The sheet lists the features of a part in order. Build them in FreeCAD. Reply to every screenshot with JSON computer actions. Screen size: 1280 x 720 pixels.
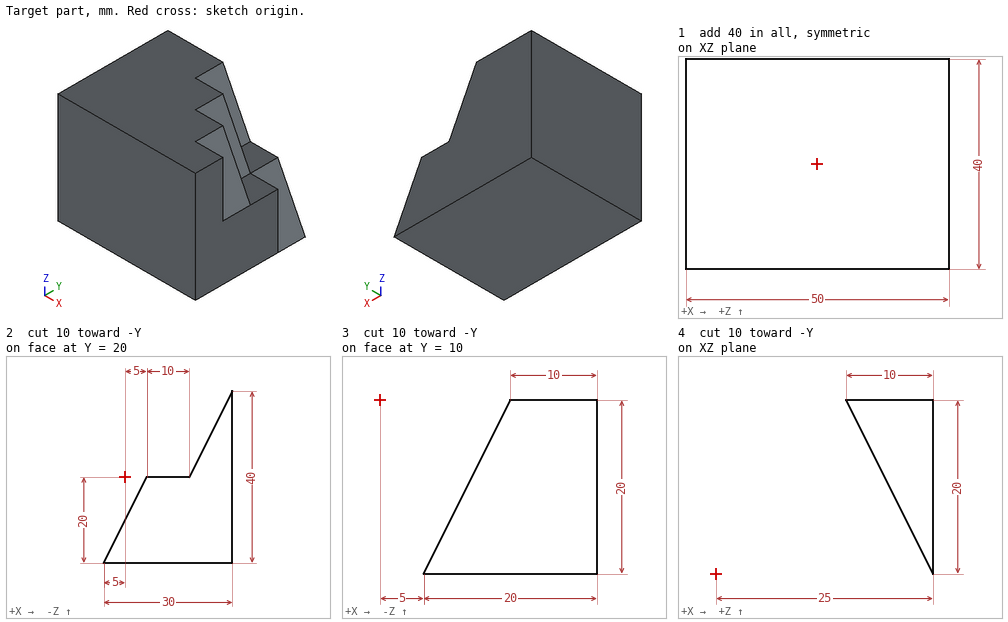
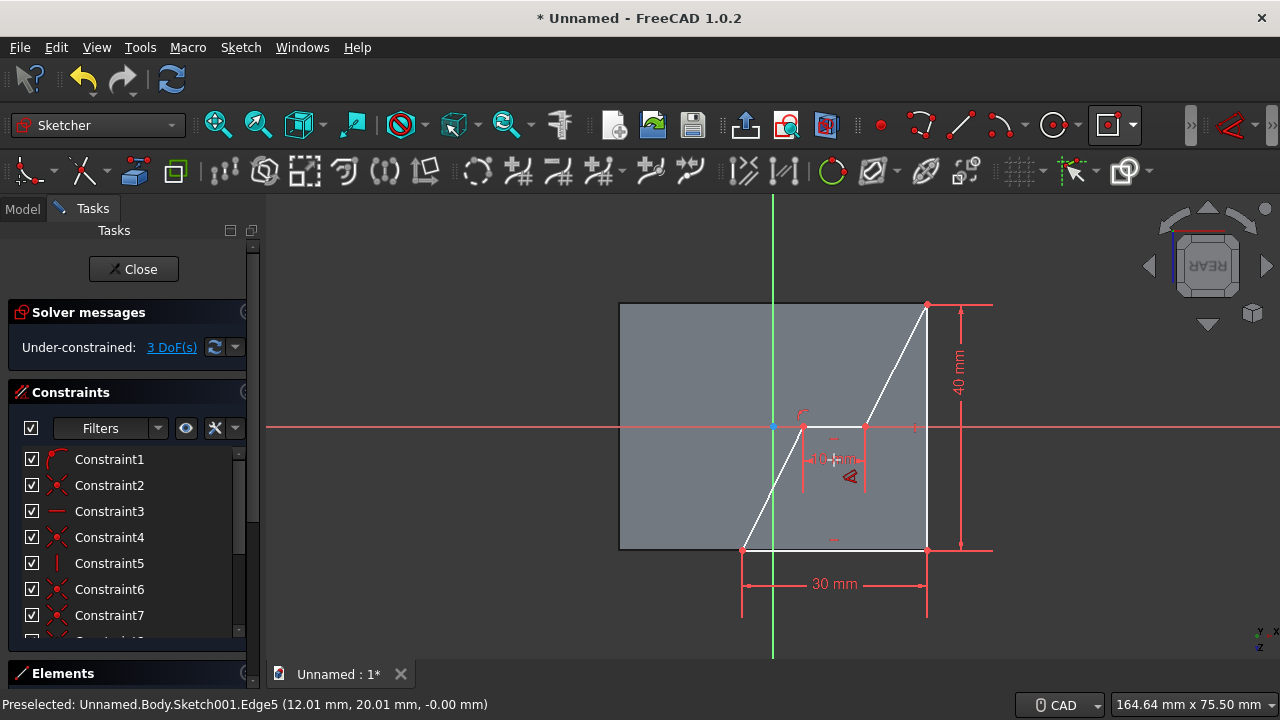
{"action": "scroll", "coordinate": [803, 426], "scroll_direction": "up", "scroll_amount": 2}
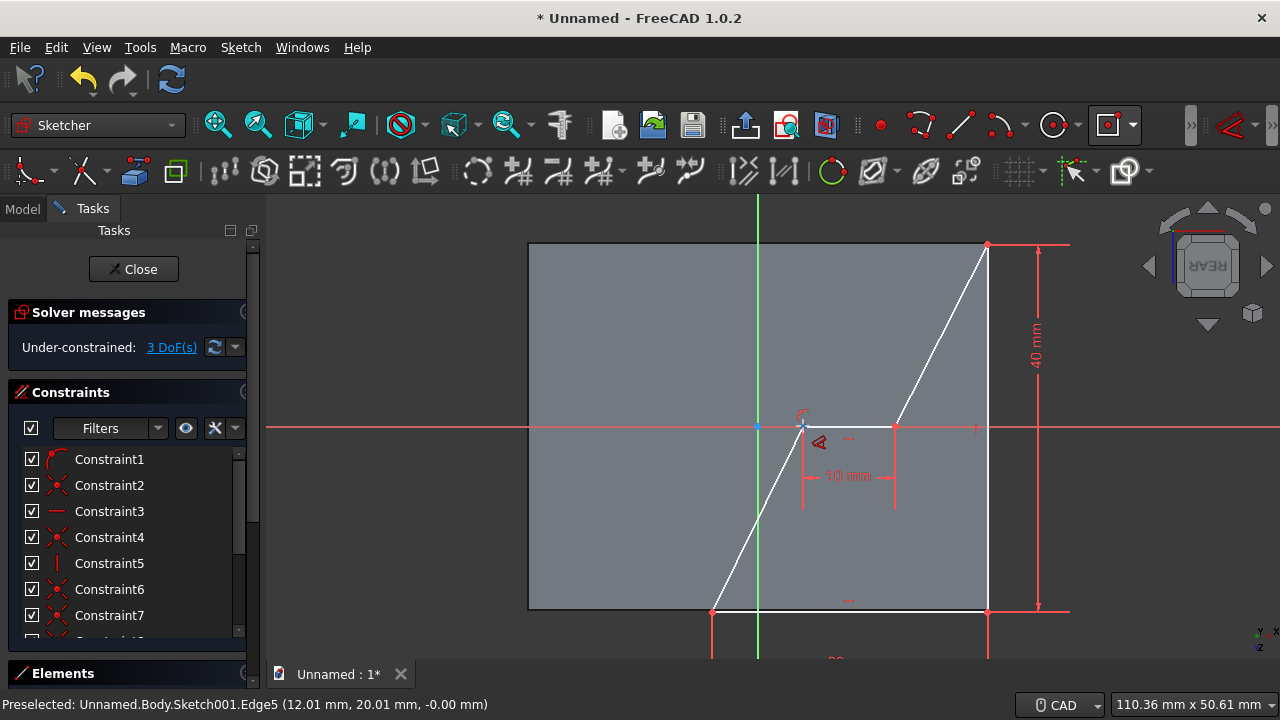
{"action": "left_click", "coordinate": [803, 426]}
{"action": "left_click", "coordinate": [781, 392]}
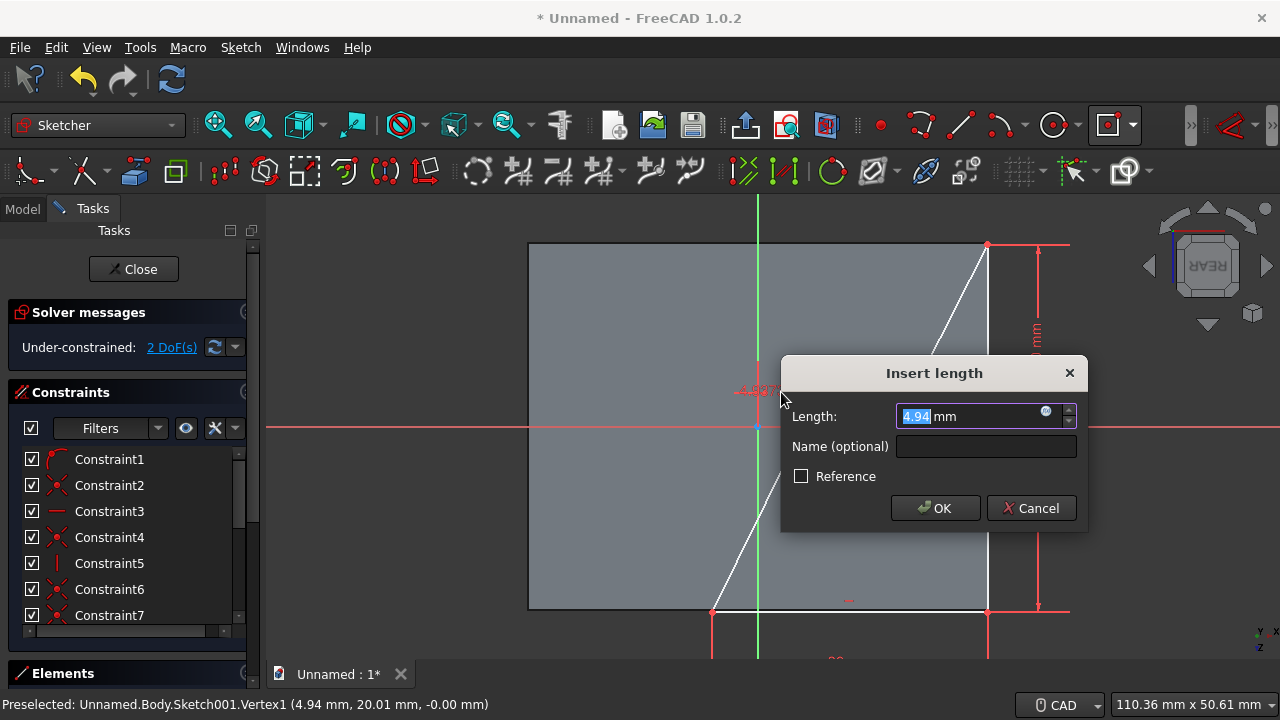
{"action": "type", "text": "5"}
{"action": "key", "text": "Return"}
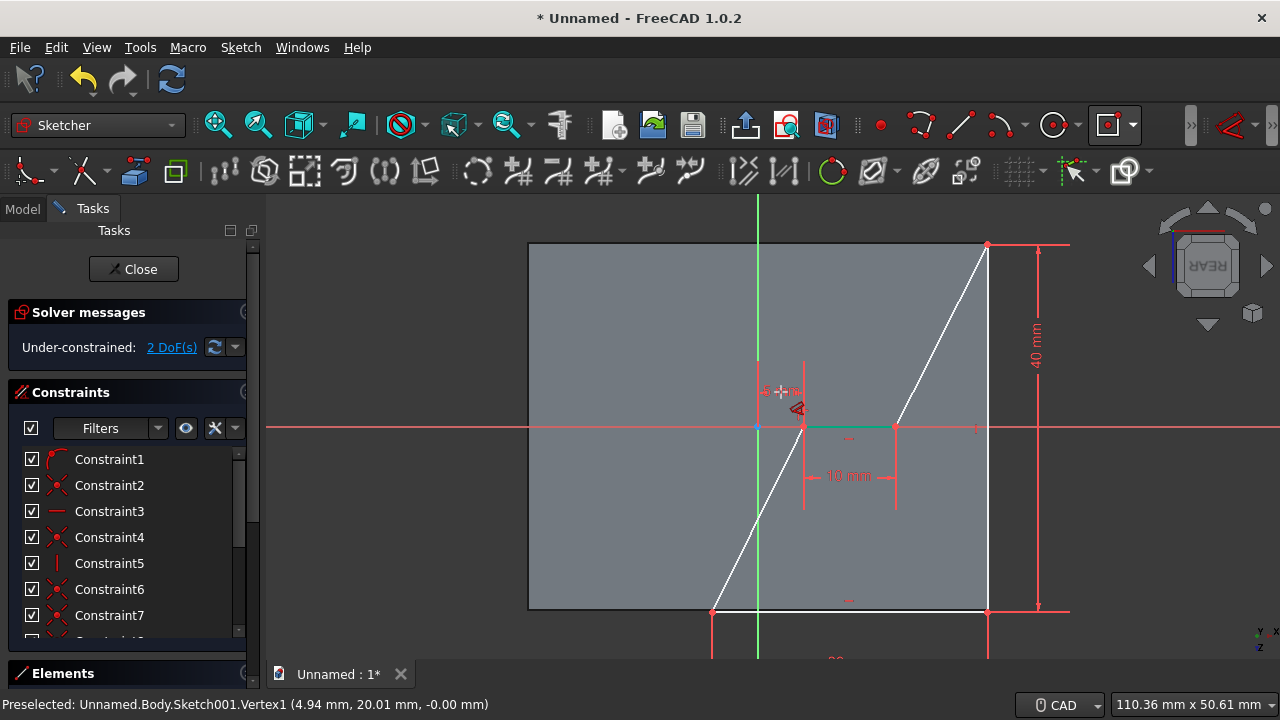
{"action": "left_click", "coordinate": [712, 612]}
{"action": "left_click", "coordinate": [735, 368]}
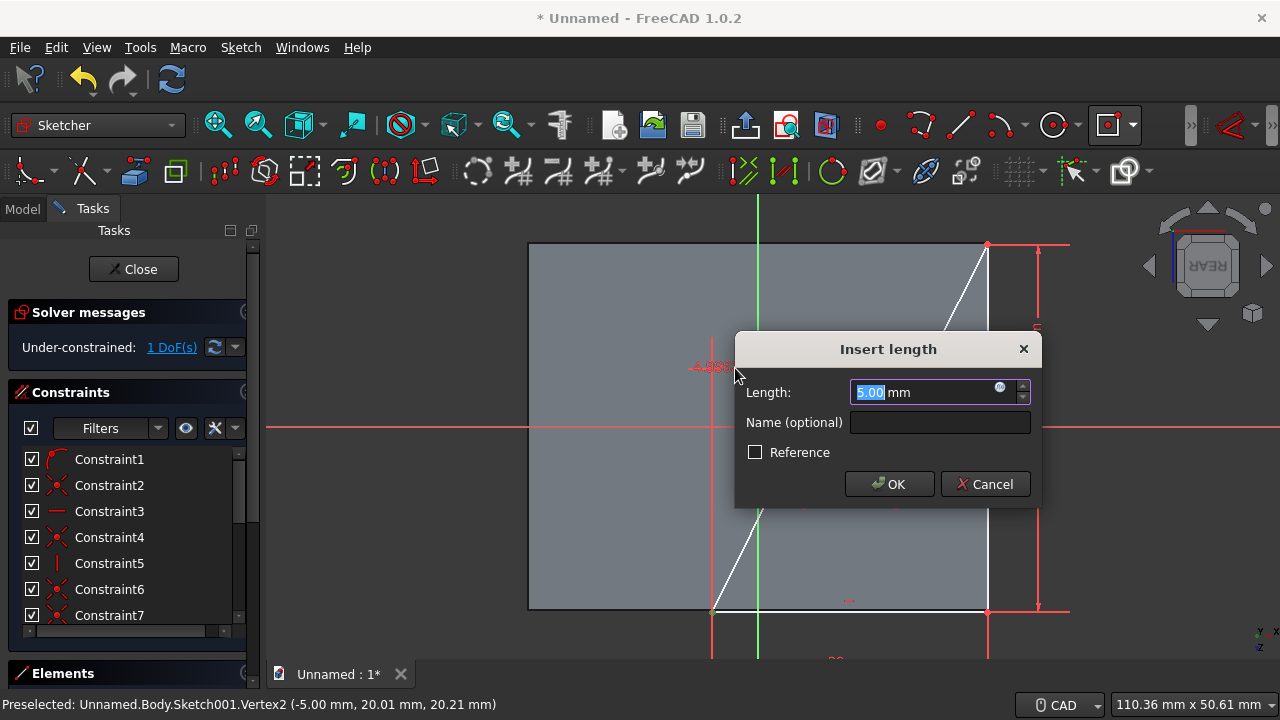
{"action": "type", "text": "5"}
{"action": "key", "text": "Return"}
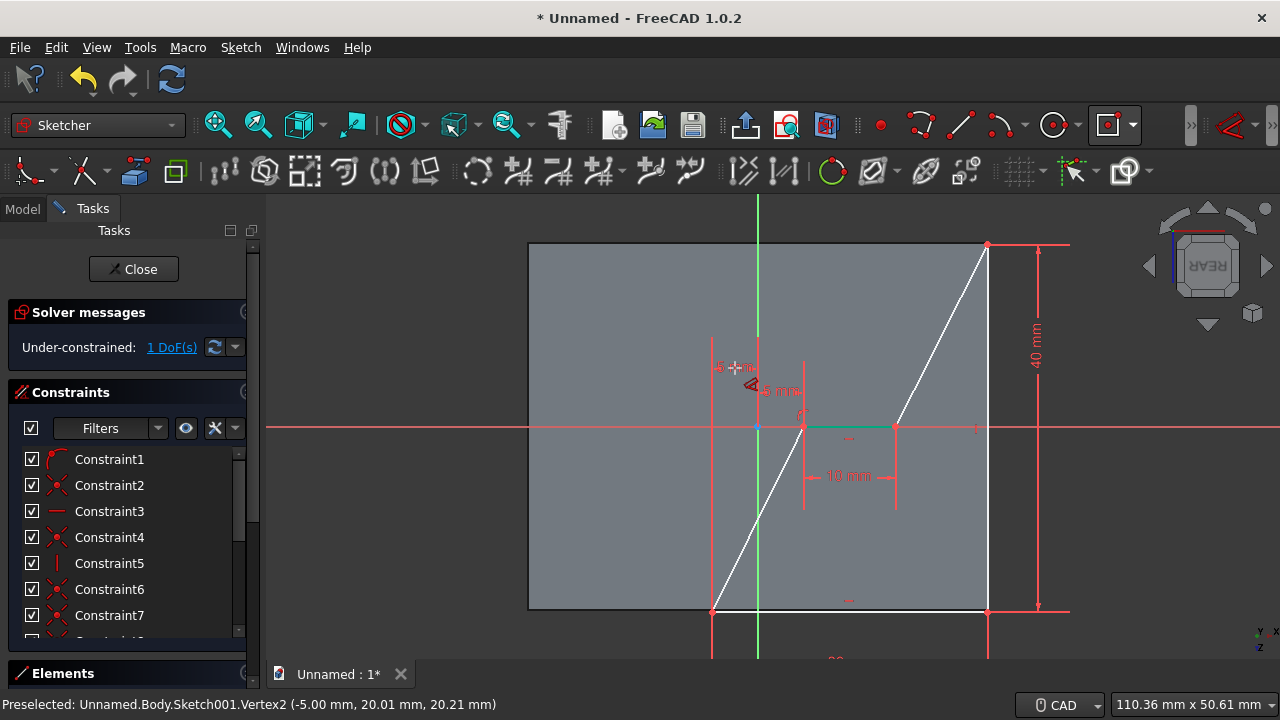
{"action": "left_click", "coordinate": [712, 612]}
{"action": "left_click", "coordinate": [678, 519]}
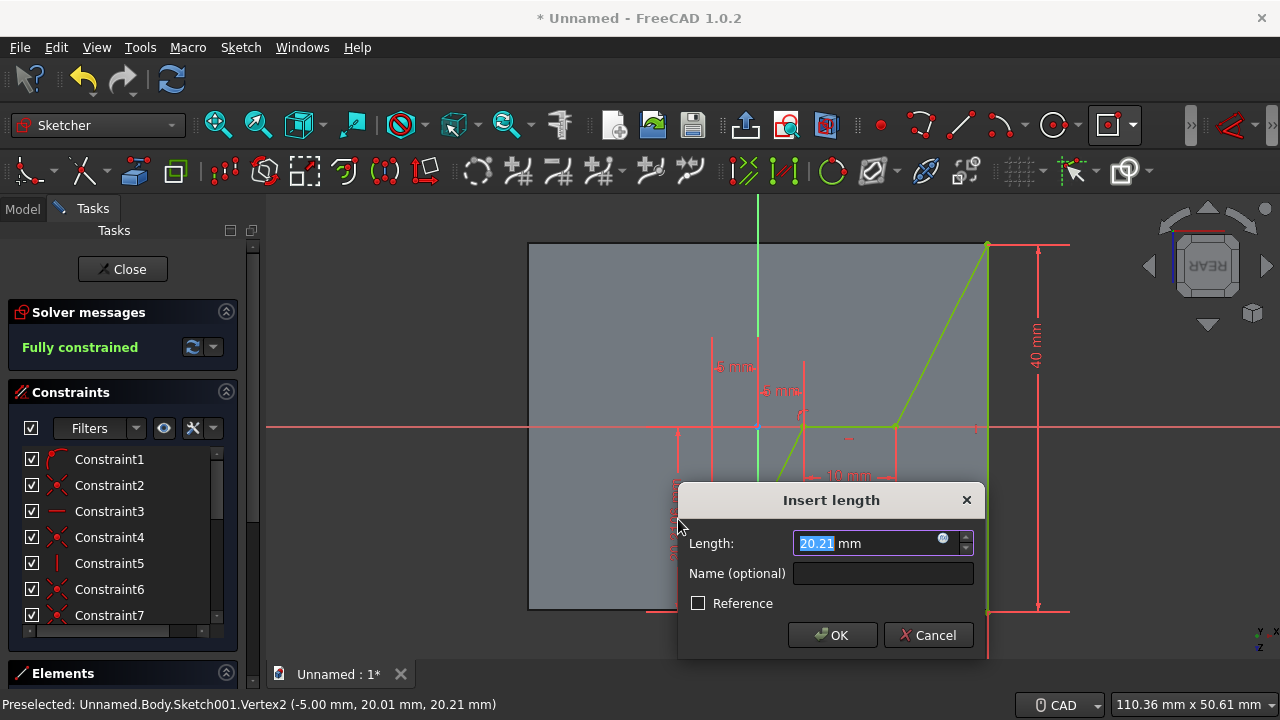
{"action": "type", "text": "20"}
{"action": "key", "text": "Return"}
{"action": "key", "text": "Escape"}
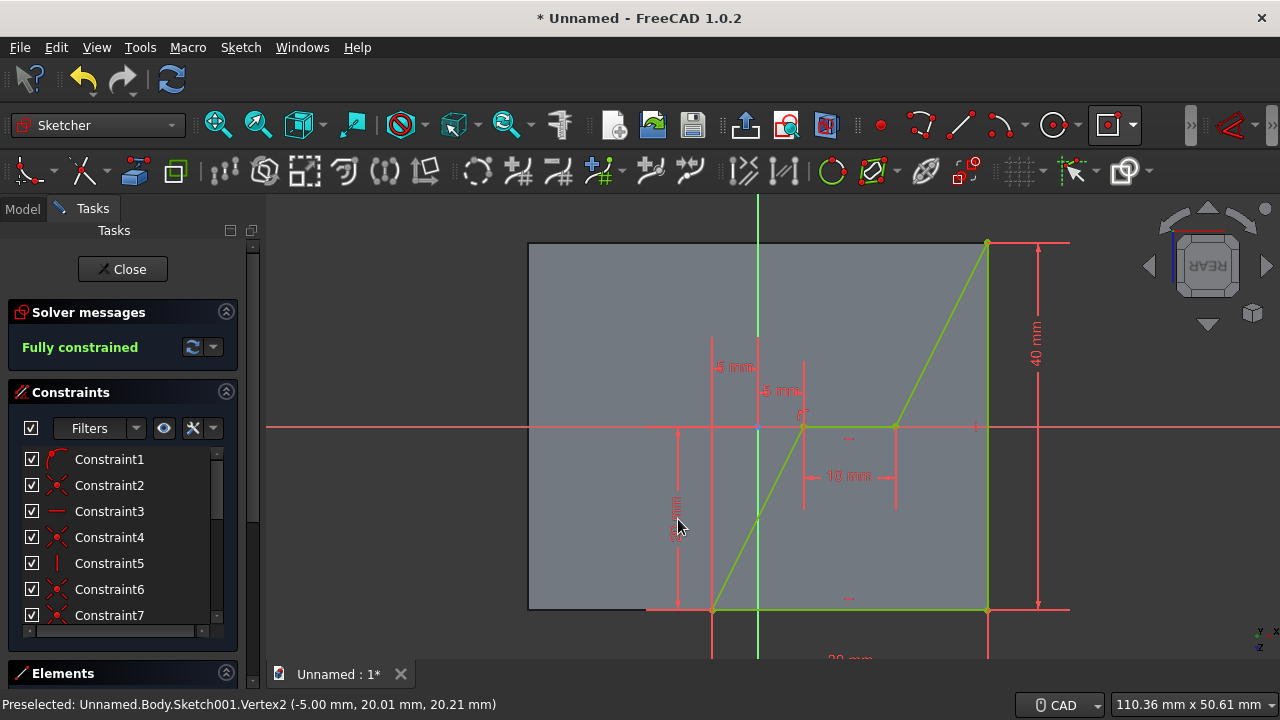
{"action": "left_click", "coordinate": [123, 269]}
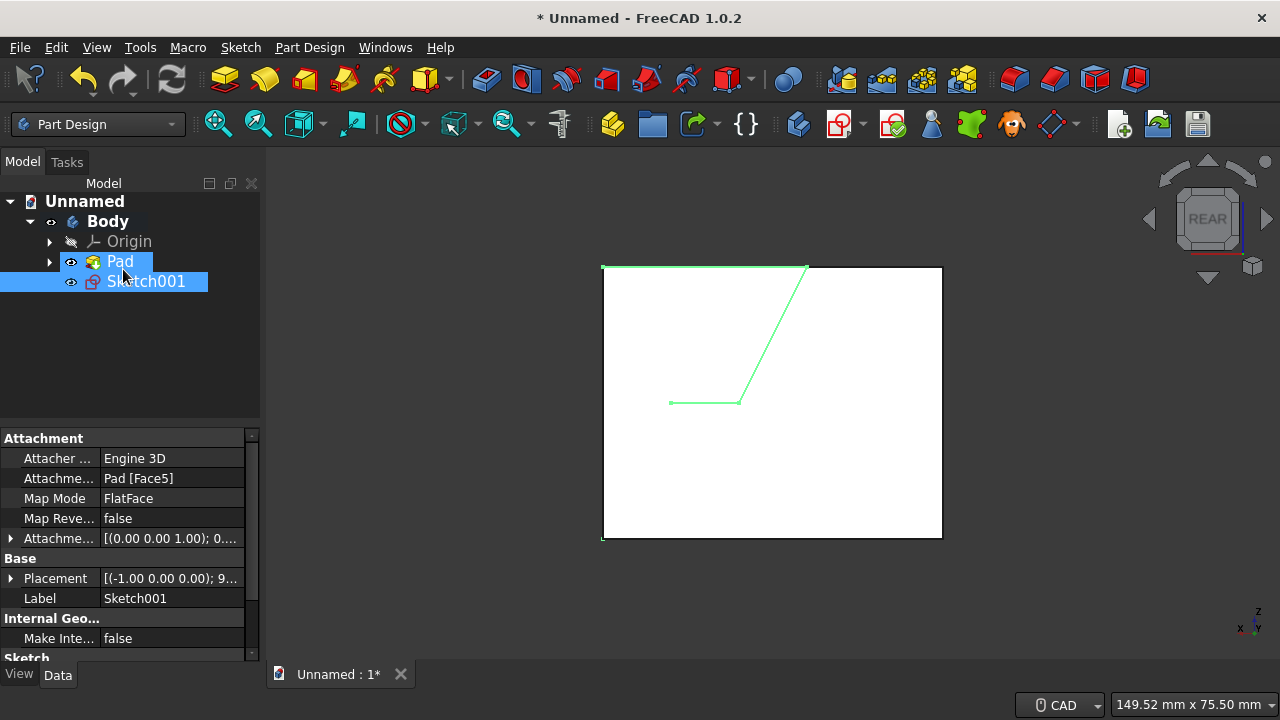
{"action": "left_click", "coordinate": [488, 80]}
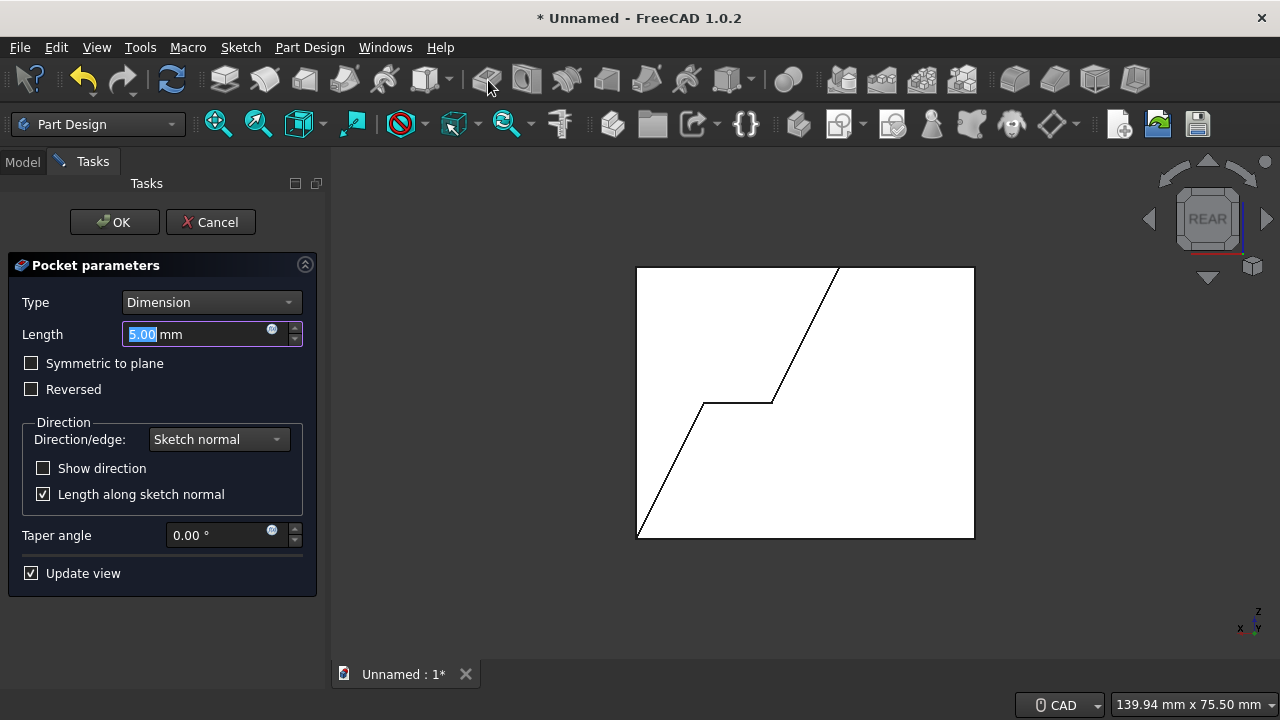
{"action": "type", "text": "10"}
{"action": "key", "text": "Tab"}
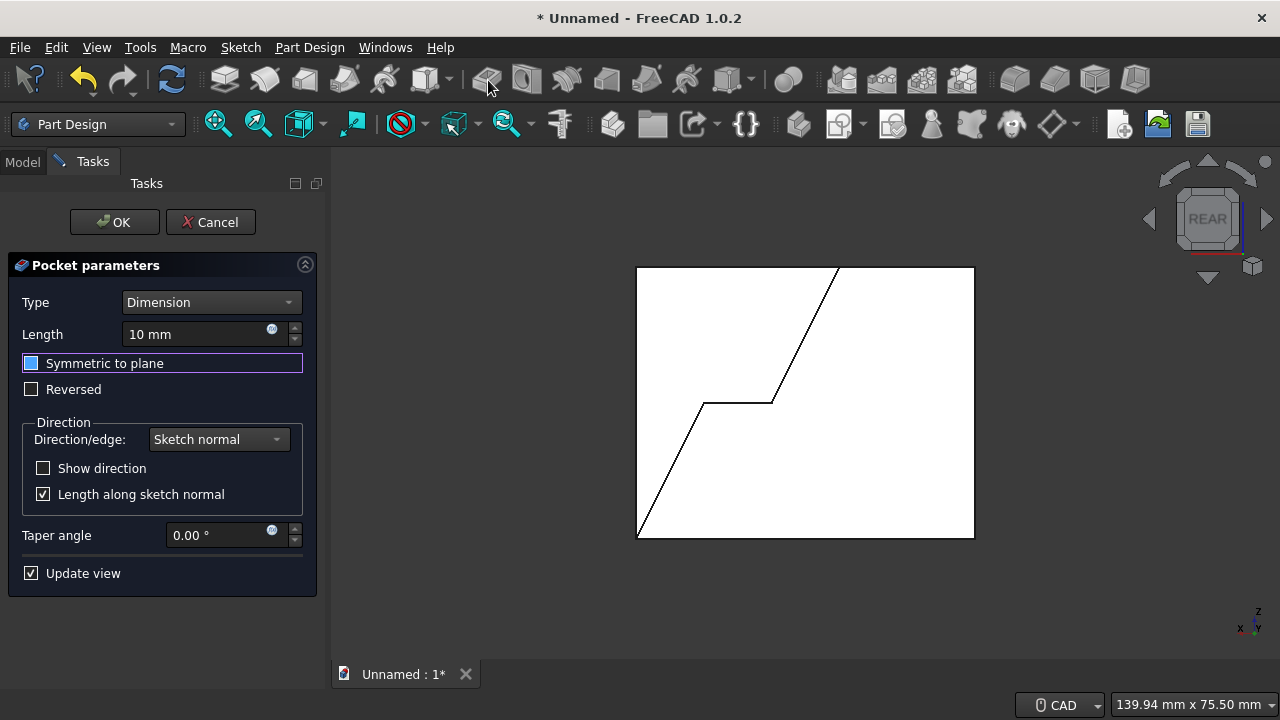
{"action": "left_click", "coordinate": [115, 222]}